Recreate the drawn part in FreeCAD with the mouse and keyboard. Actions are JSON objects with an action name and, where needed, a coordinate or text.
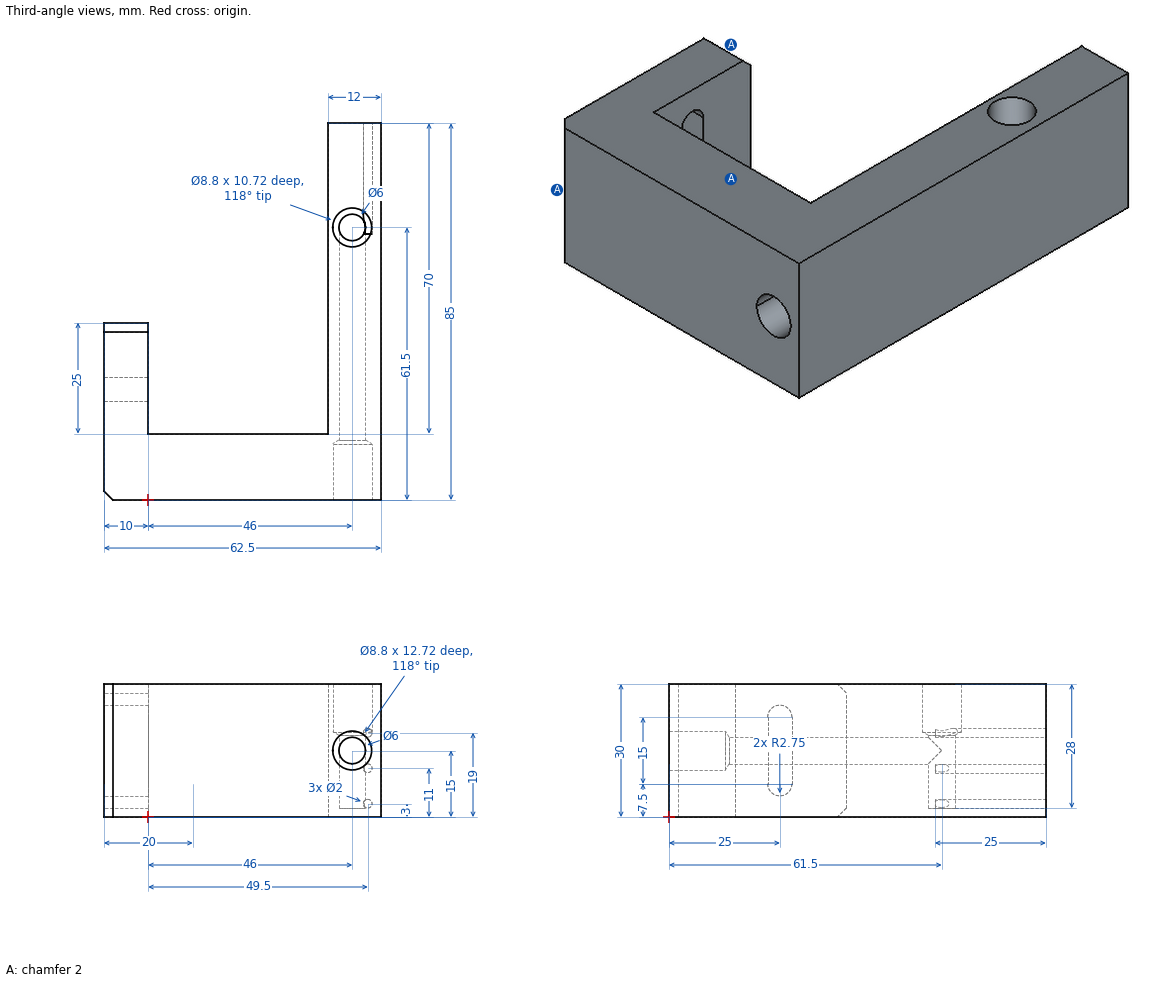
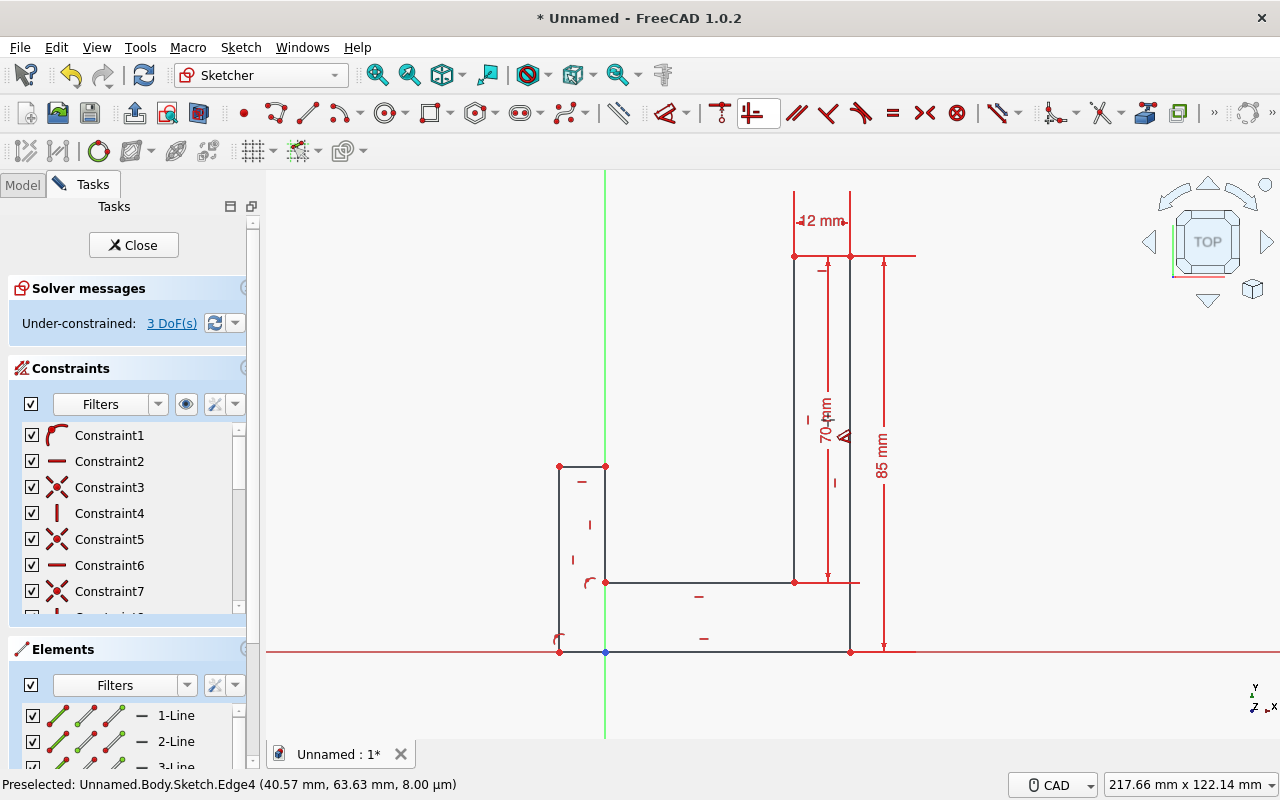
{"action": "left_click", "coordinate": [605, 548]}
{"action": "left_click", "coordinate": [639, 525]}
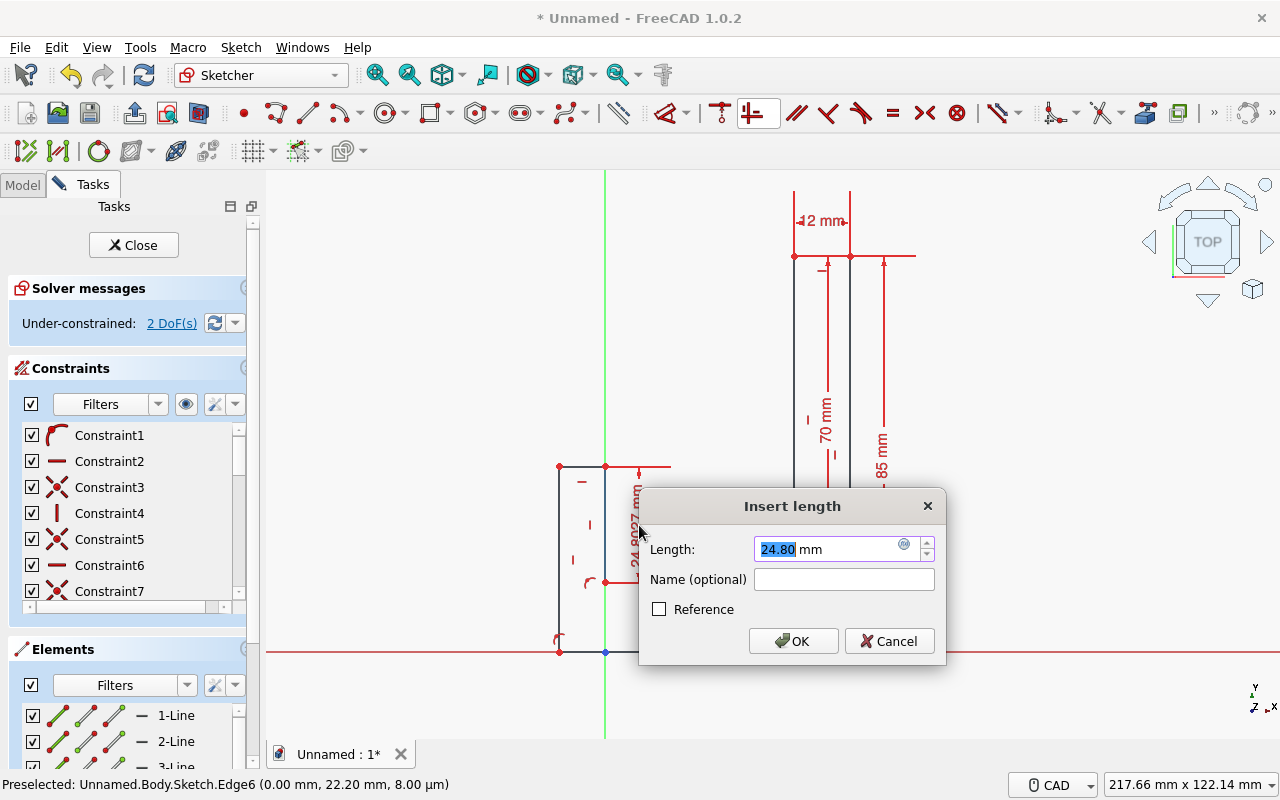
{"action": "type", "text": "25"}
{"action": "key", "text": "Return"}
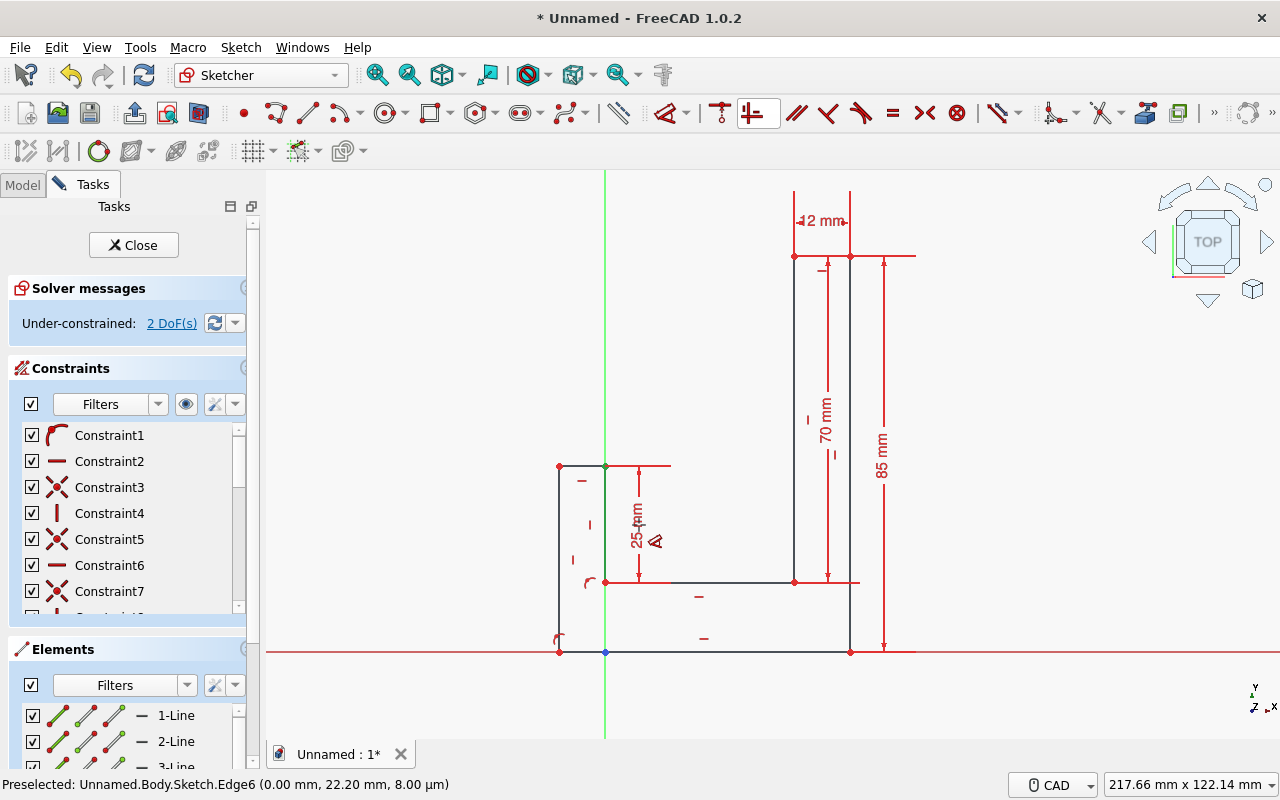
{"action": "left_click", "coordinate": [591, 466]}
{"action": "left_click", "coordinate": [582, 500]}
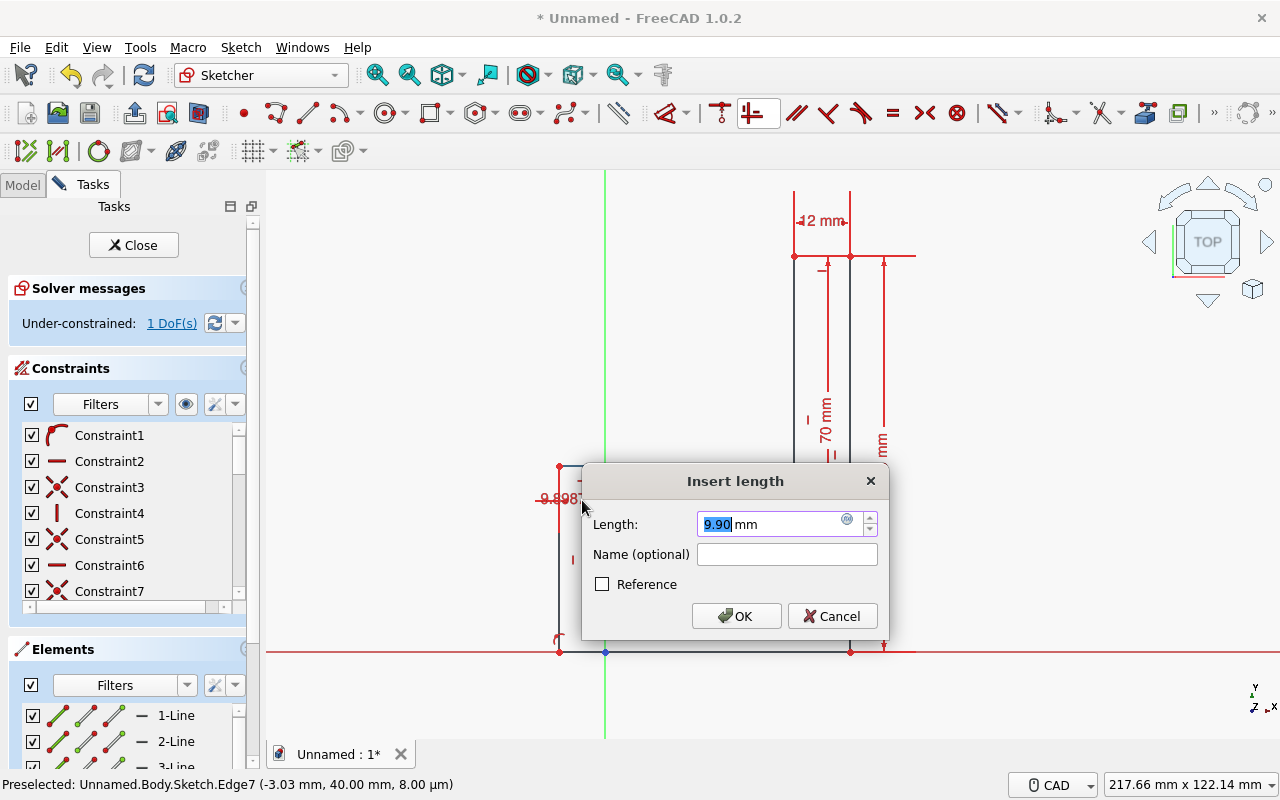
{"action": "type", "text": "10"}
{"action": "key", "text": "Return"}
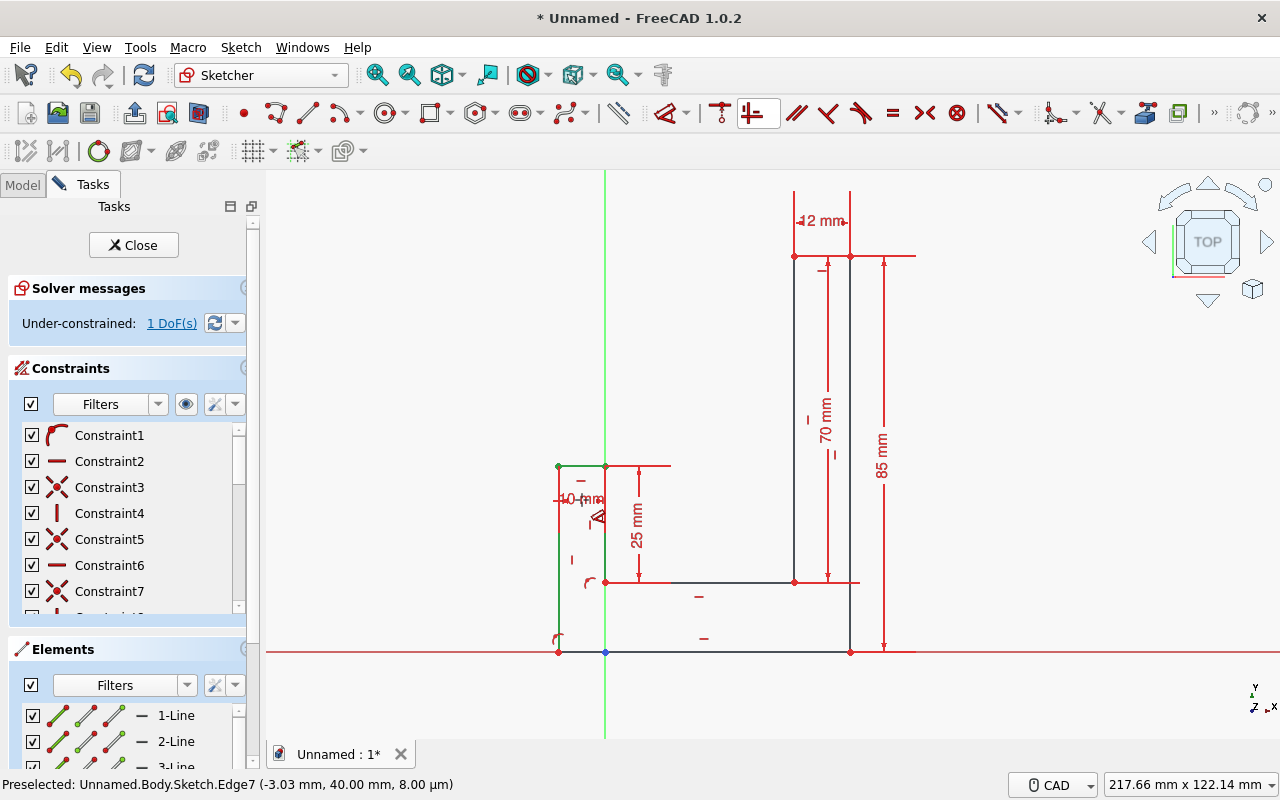
{"action": "left_click", "coordinate": [646, 652]}
{"action": "left_click", "coordinate": [704, 686]}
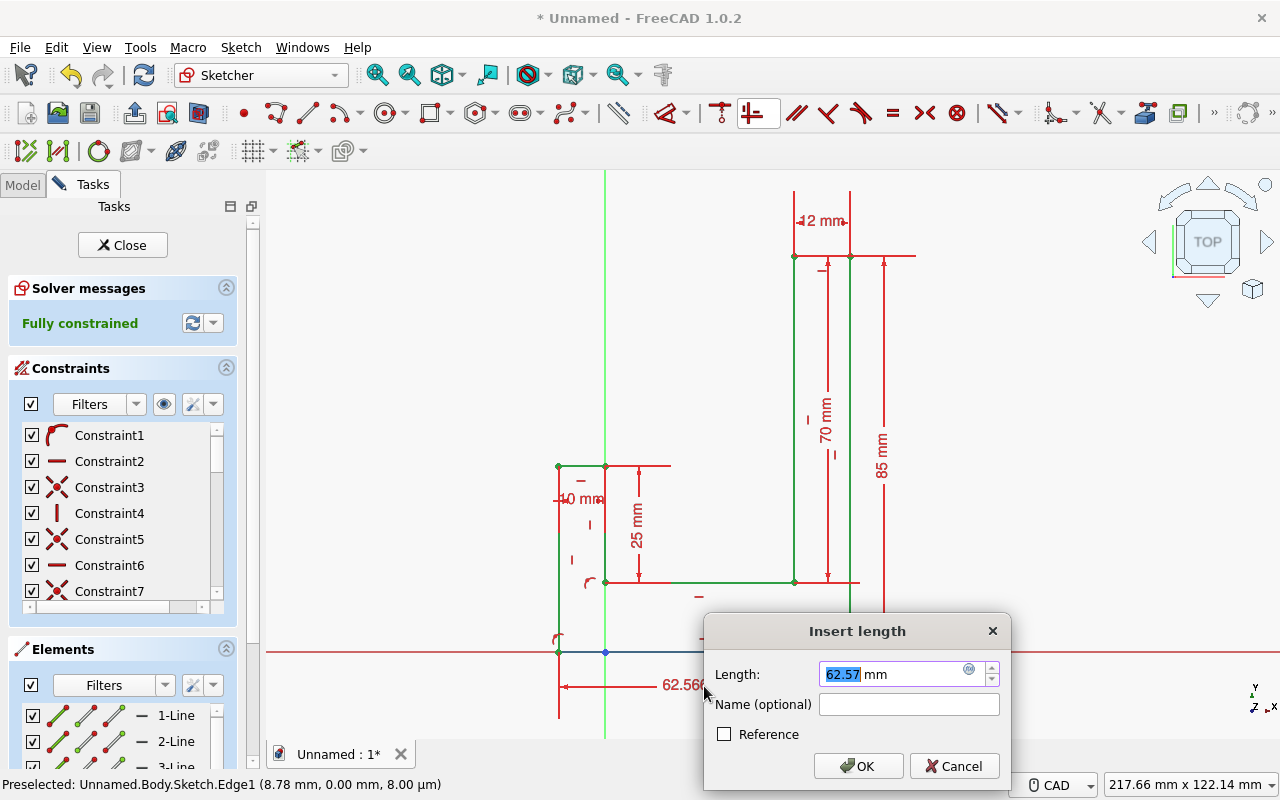
{"action": "type", "text": "62.5"}
{"action": "key", "text": "Return"}
{"action": "key", "text": "Escape"}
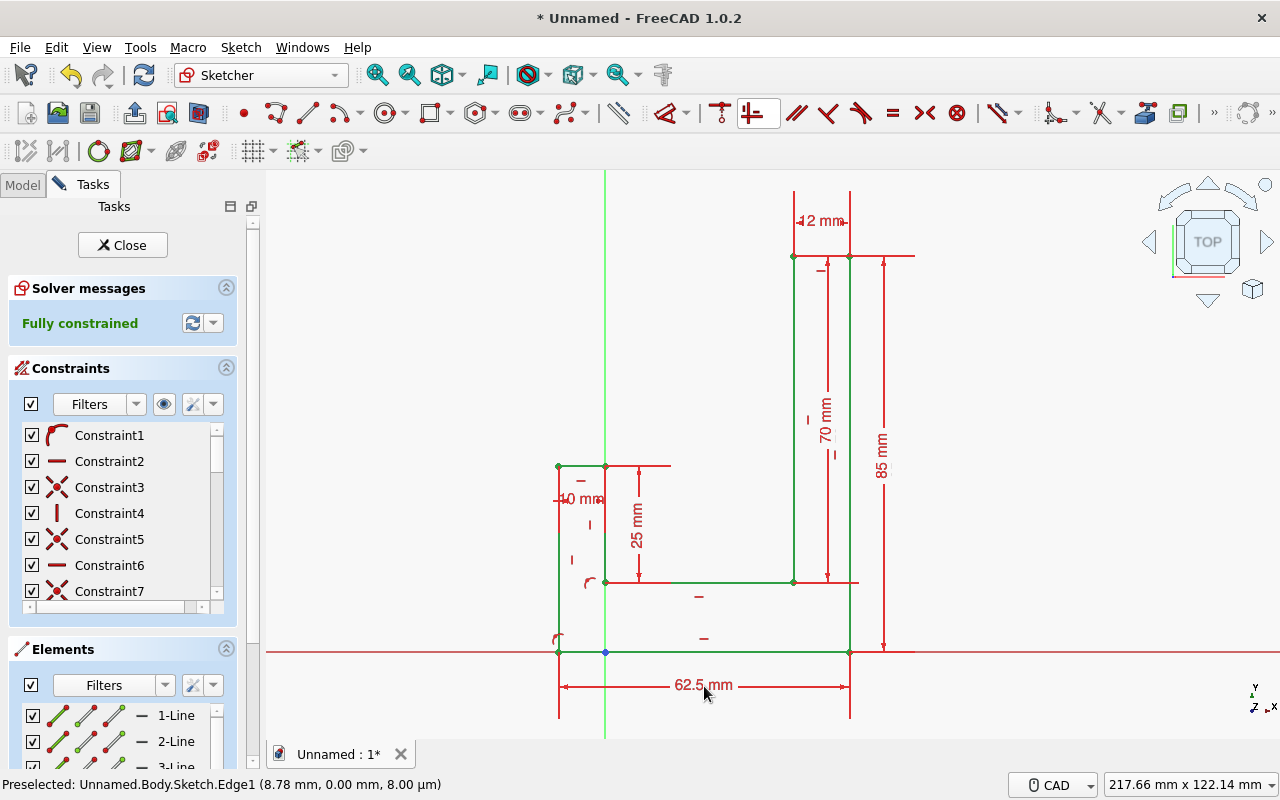
{"action": "left_click", "coordinate": [123, 245]}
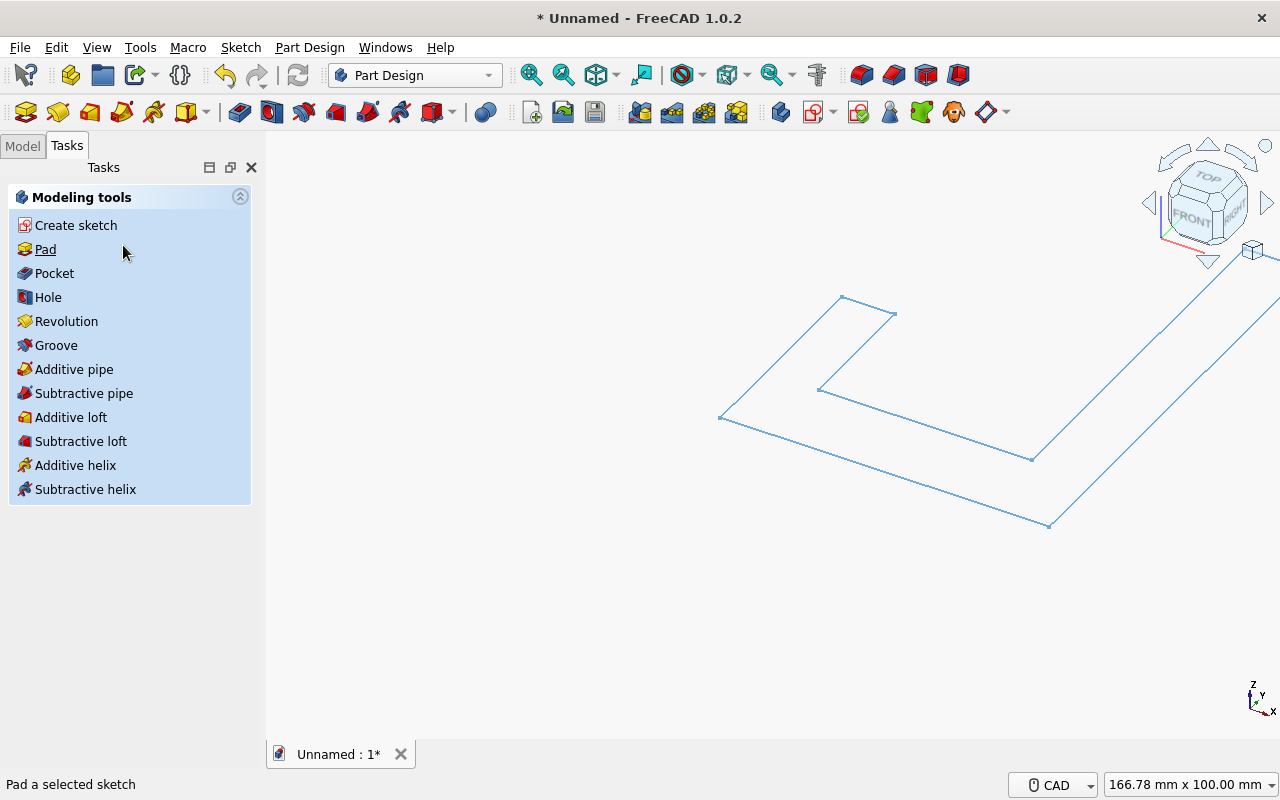
{"action": "left_click", "coordinate": [26, 112]}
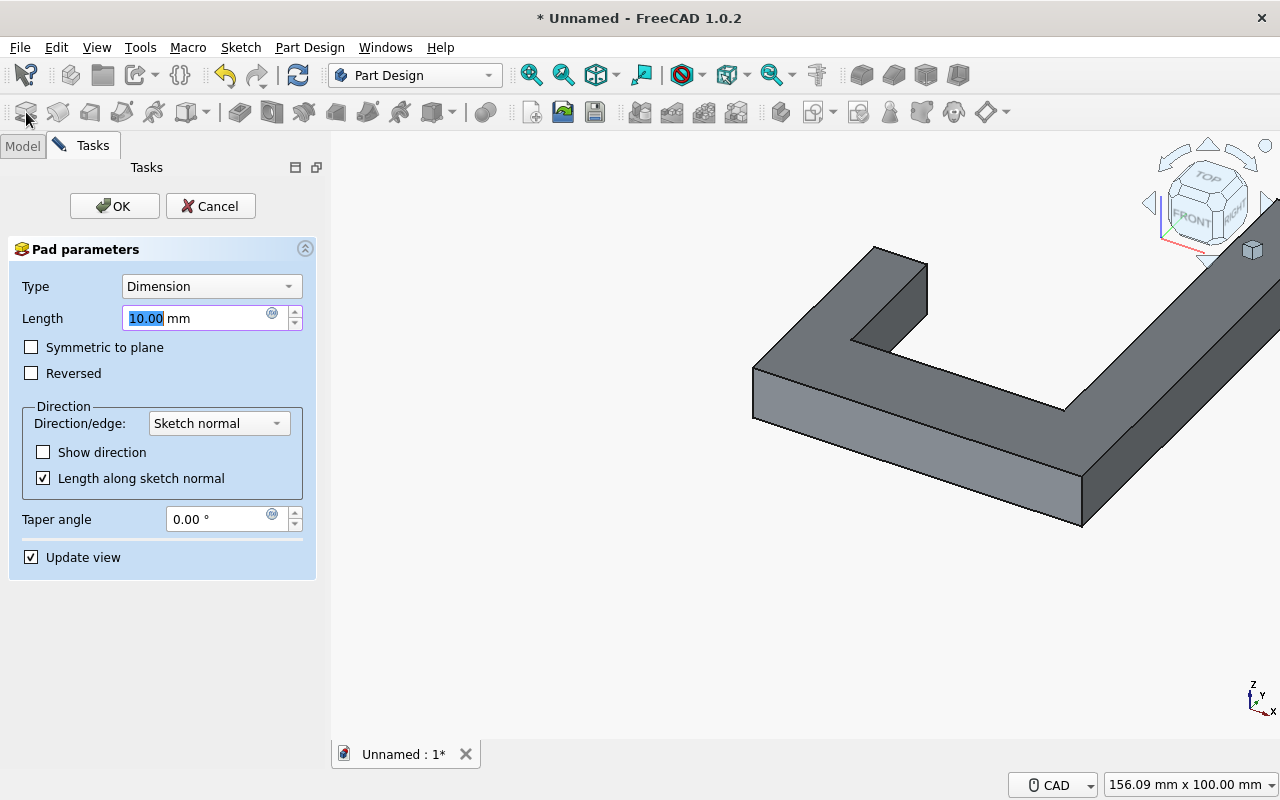
{"action": "type", "text": "30"}
{"action": "key", "text": "Tab"}